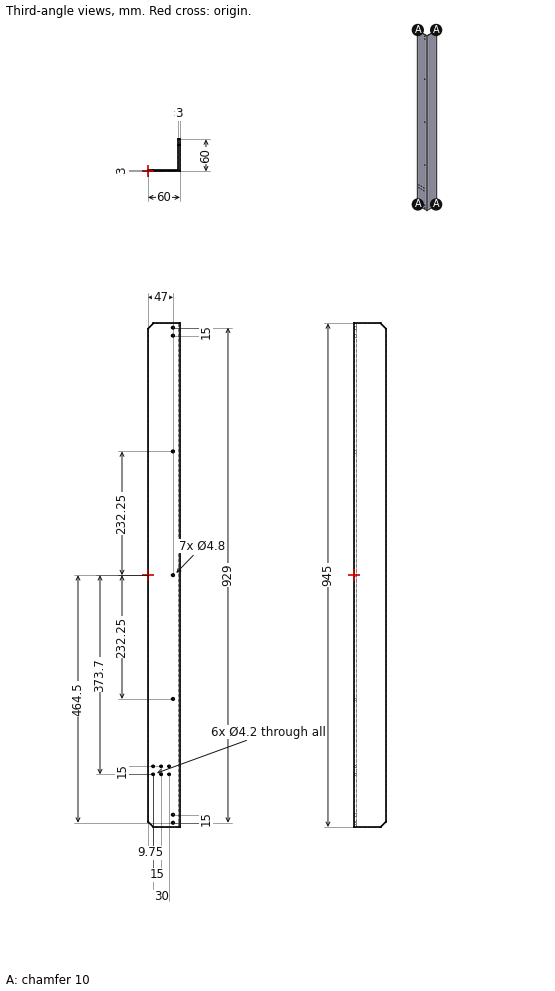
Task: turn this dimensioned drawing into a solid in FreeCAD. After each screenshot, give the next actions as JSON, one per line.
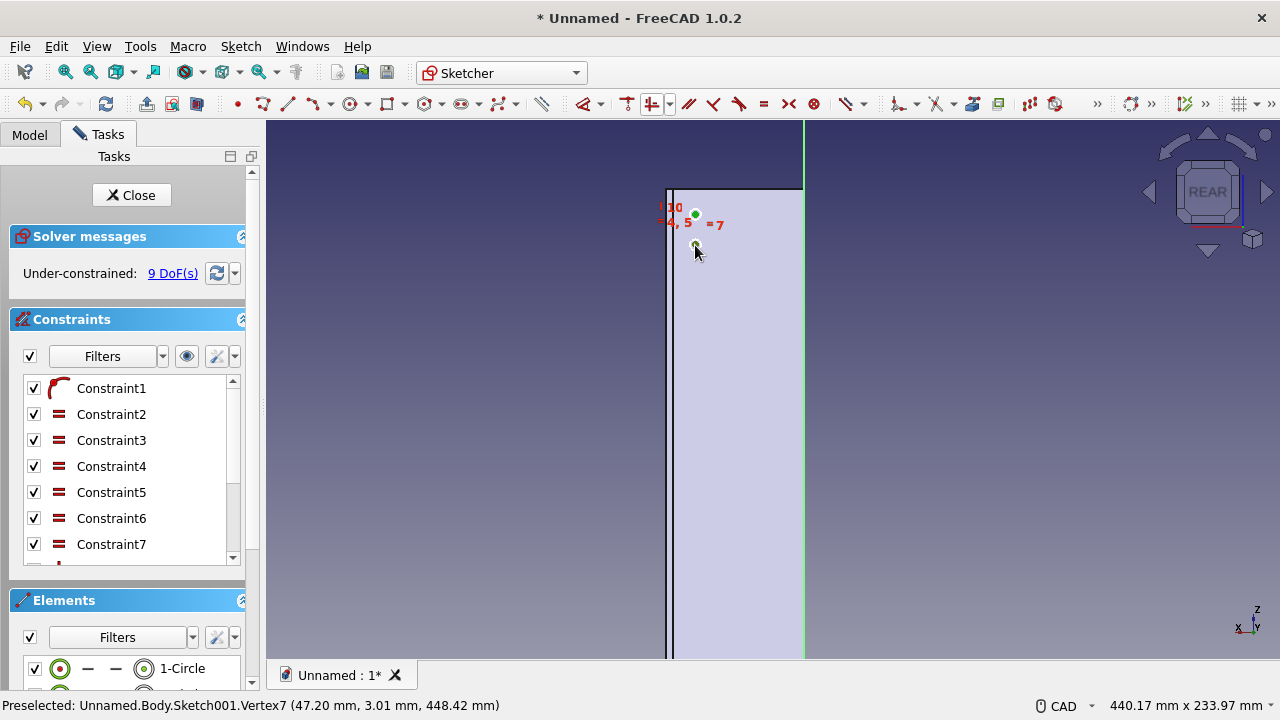
{"action": "key", "text": "v"}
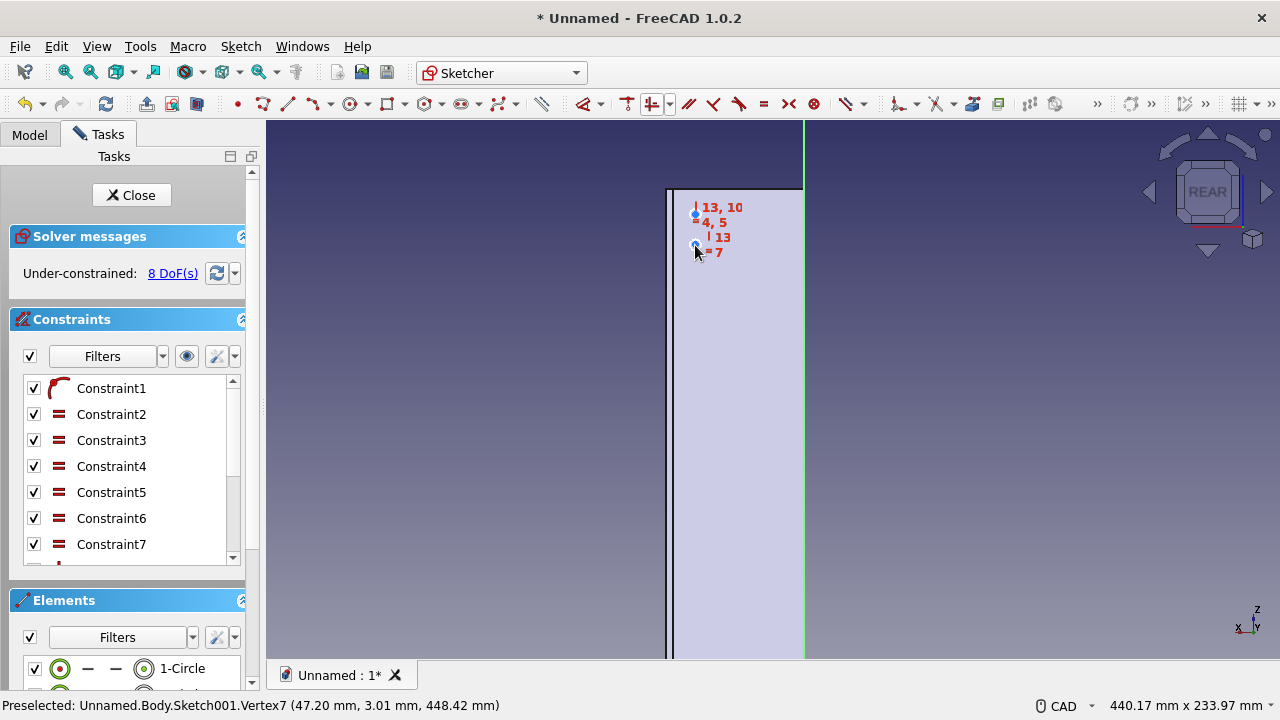
{"action": "left_click", "coordinate": [582, 104]}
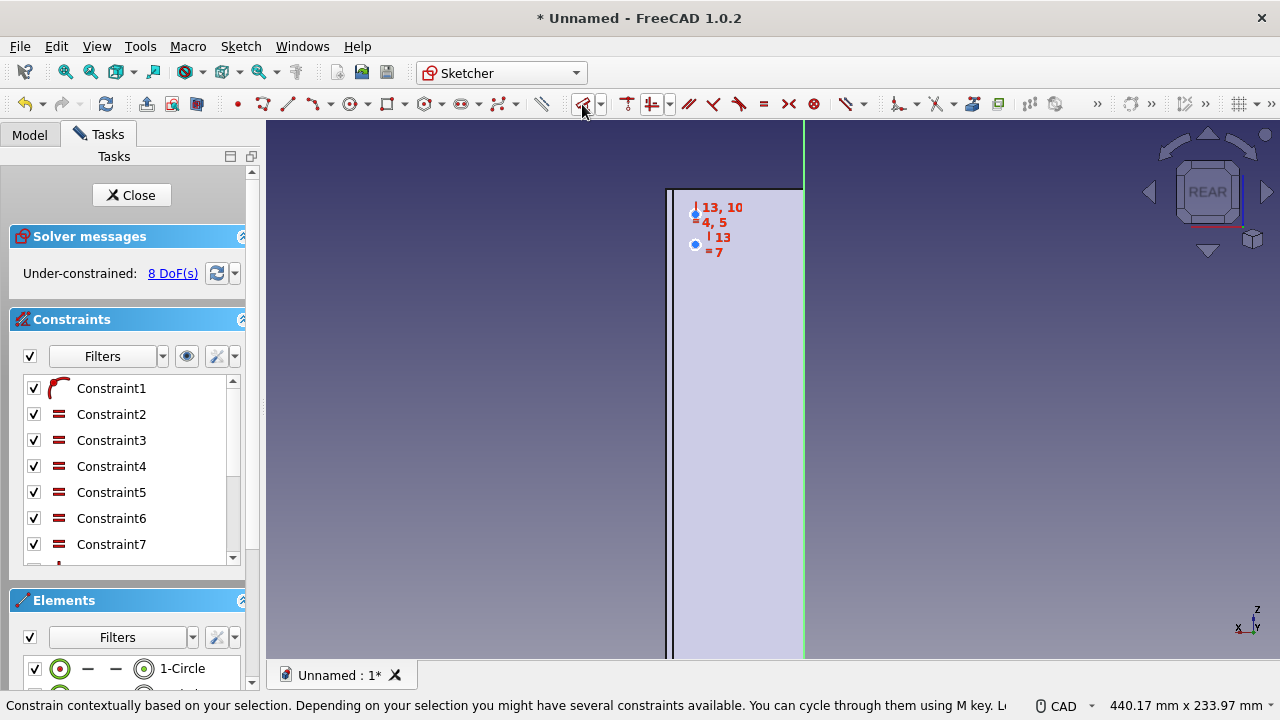
{"action": "scroll", "coordinate": [696, 214], "scroll_direction": "down", "scroll_amount": 9}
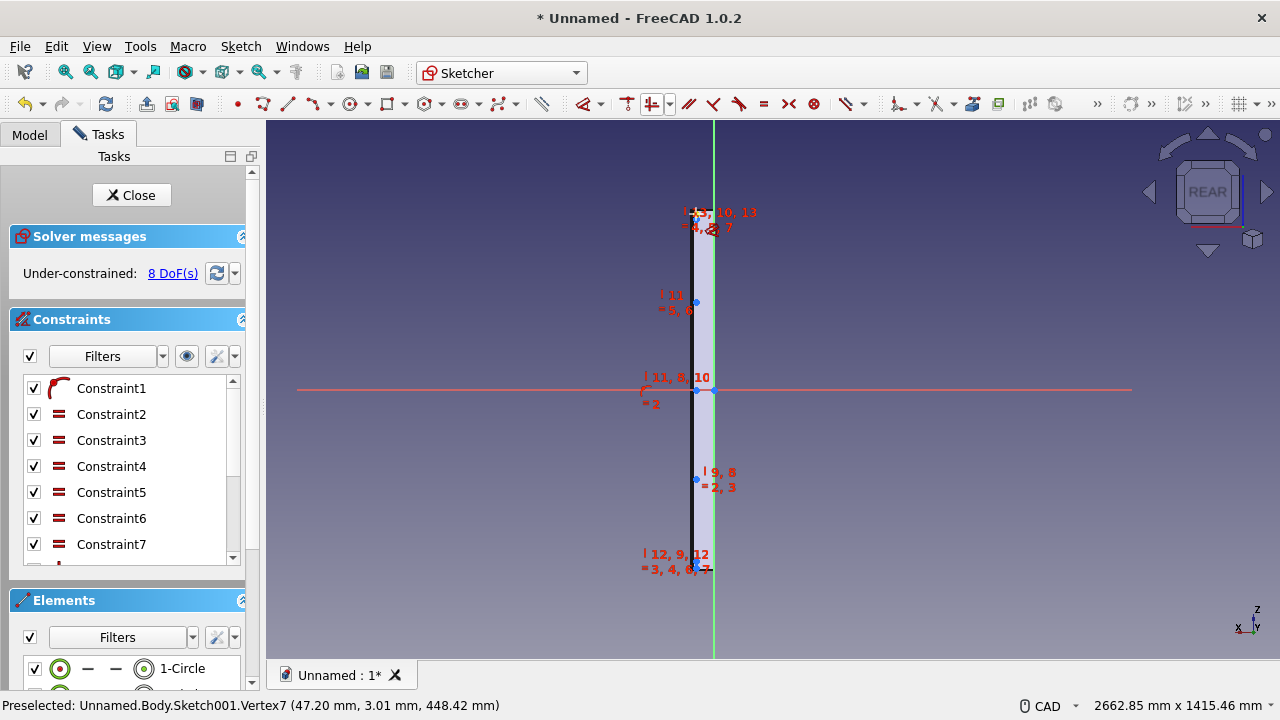
{"action": "scroll", "coordinate": [696, 391], "scroll_direction": "up", "scroll_amount": 16}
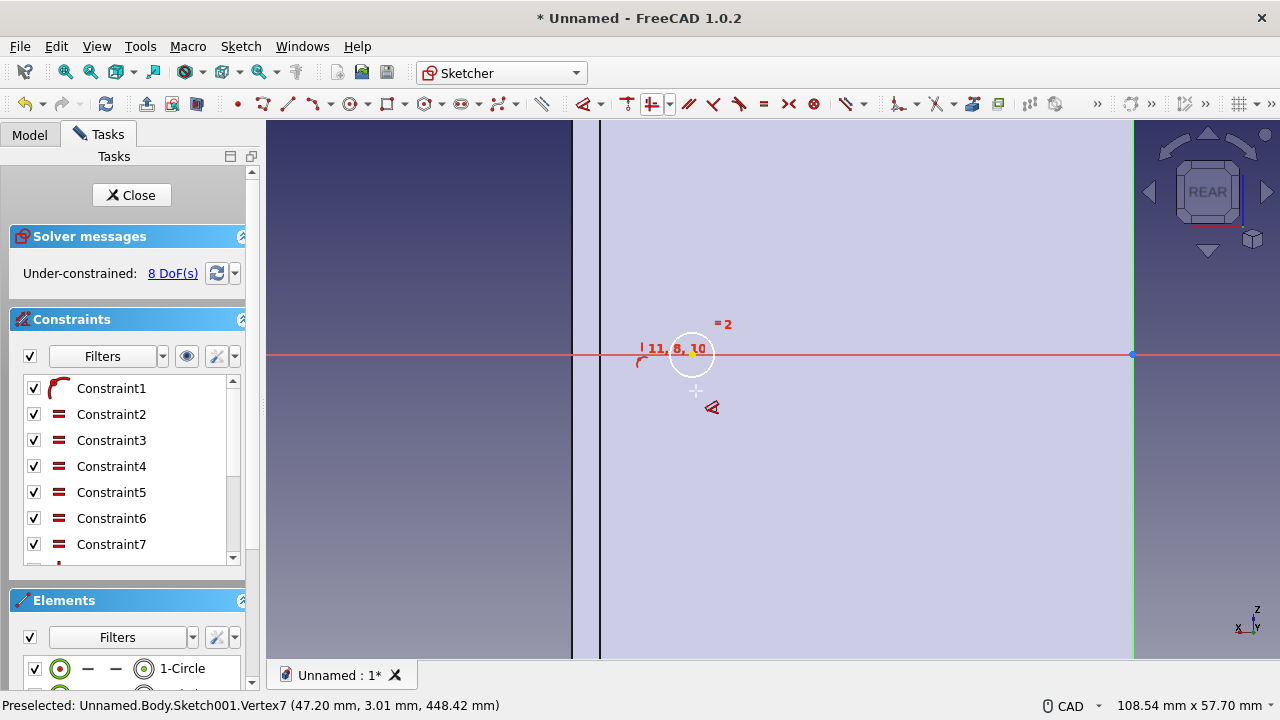
{"action": "left_click", "coordinate": [677, 371]}
{"action": "left_click", "coordinate": [655, 394]}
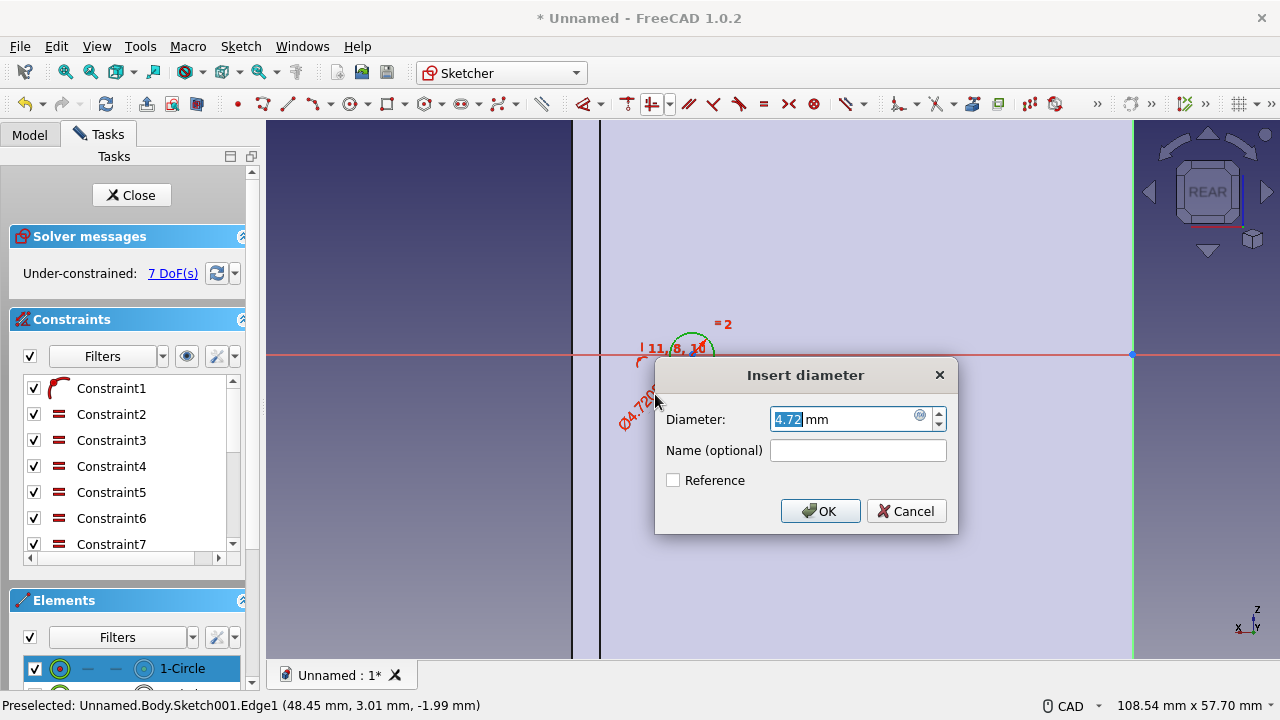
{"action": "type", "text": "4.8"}
{"action": "key", "text": "Return"}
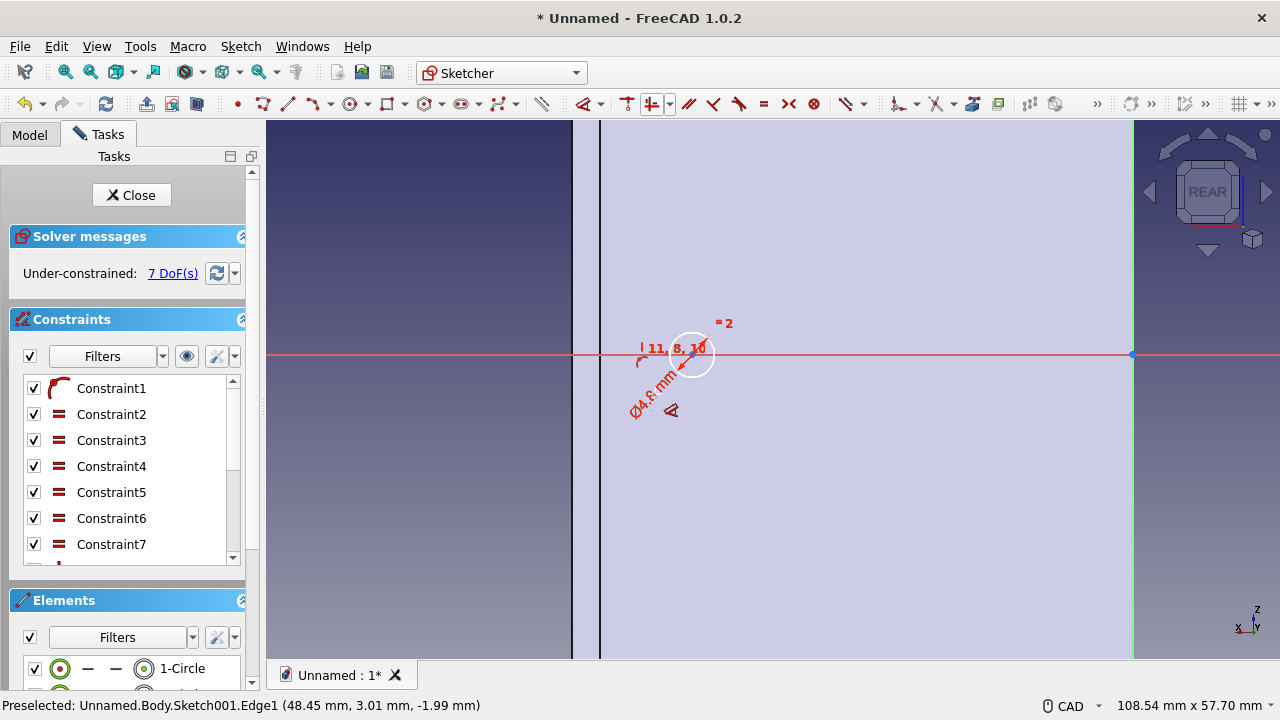
{"action": "scroll", "coordinate": [696, 391], "scroll_direction": "down", "scroll_amount": 16}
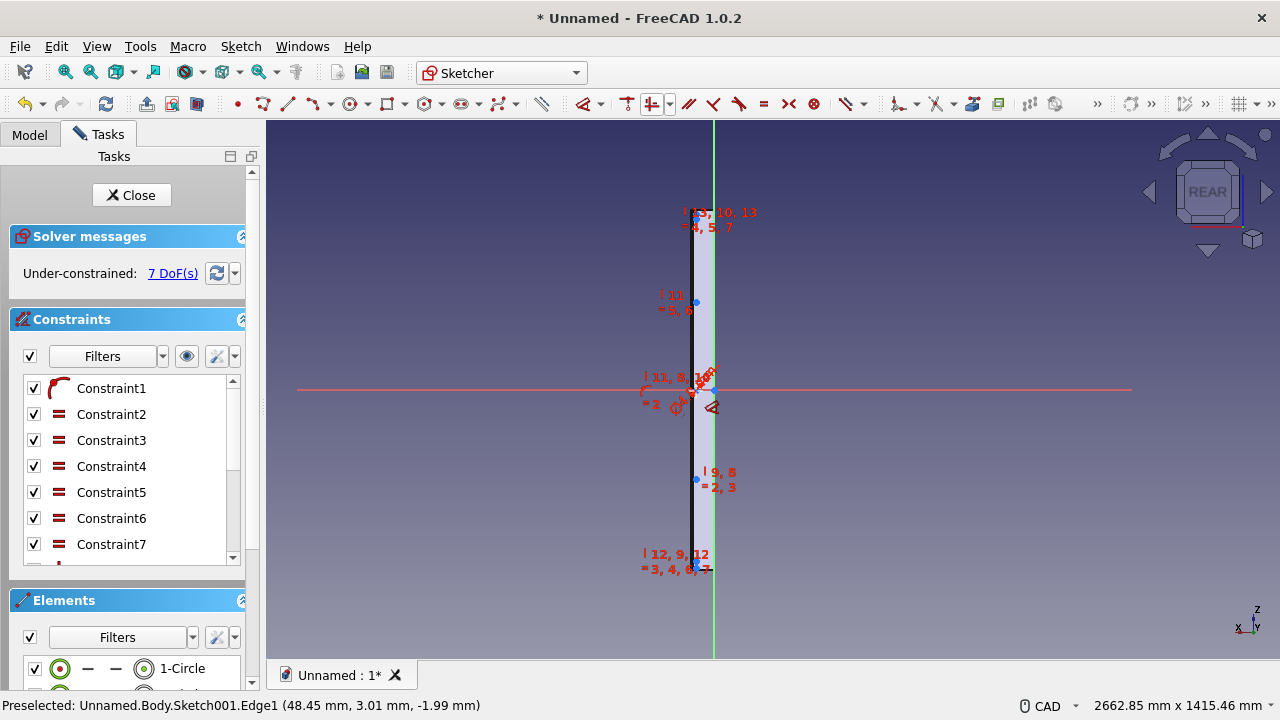
{"action": "scroll", "coordinate": [696, 390], "scroll_direction": "up", "scroll_amount": 4}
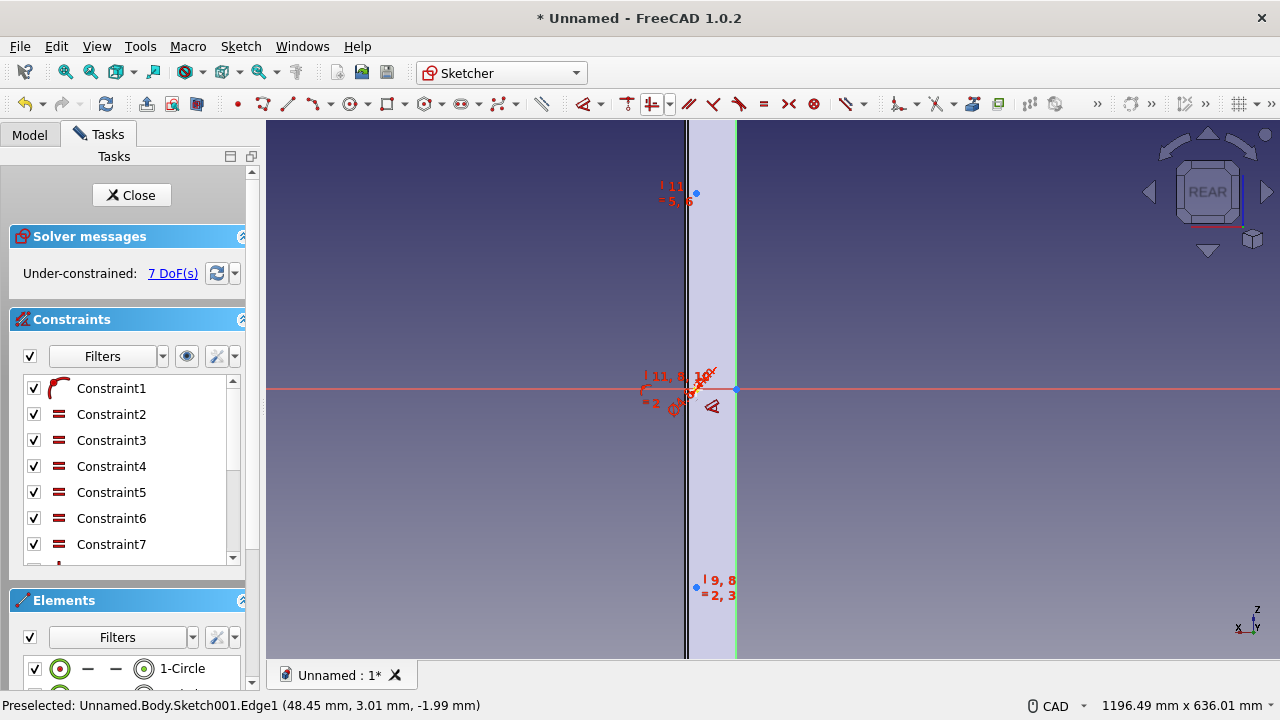
{"action": "left_click", "coordinate": [696, 389]}
{"action": "left_click", "coordinate": [716, 423]}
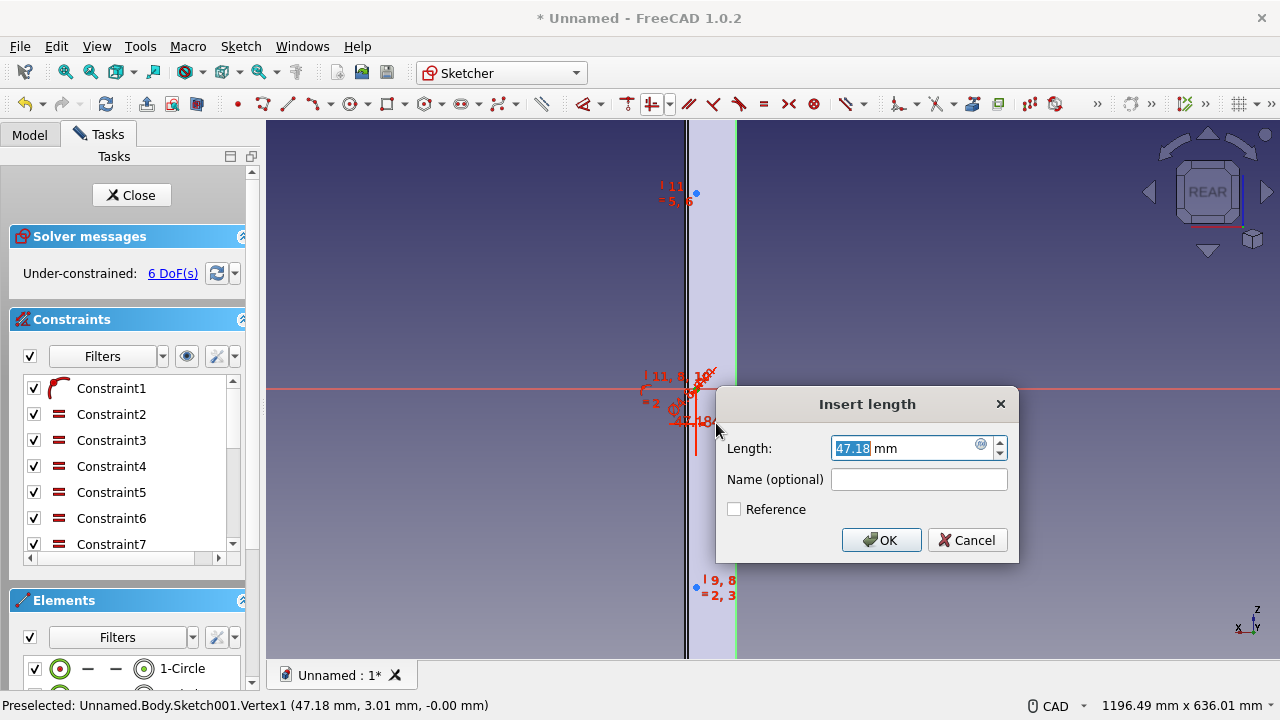
{"action": "type", "text": "47"}
{"action": "key", "text": "Return"}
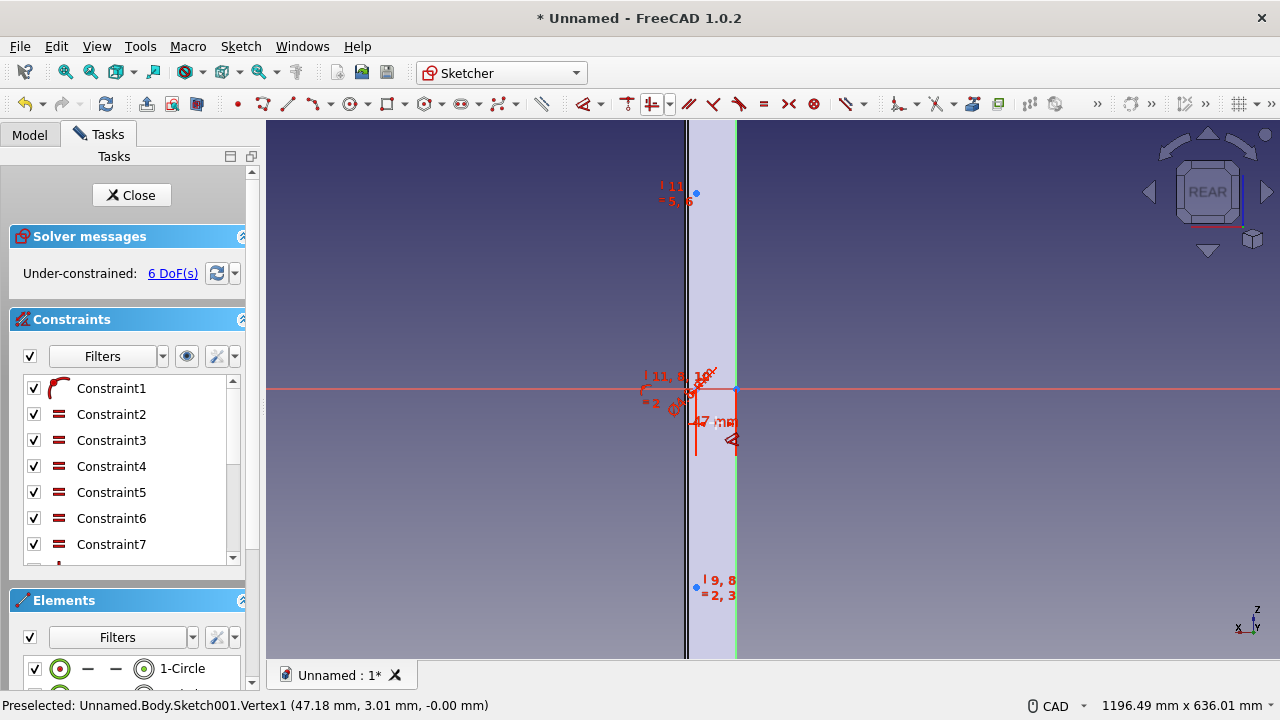
{"action": "scroll", "coordinate": [696, 390], "scroll_direction": "down", "scroll_amount": 4}